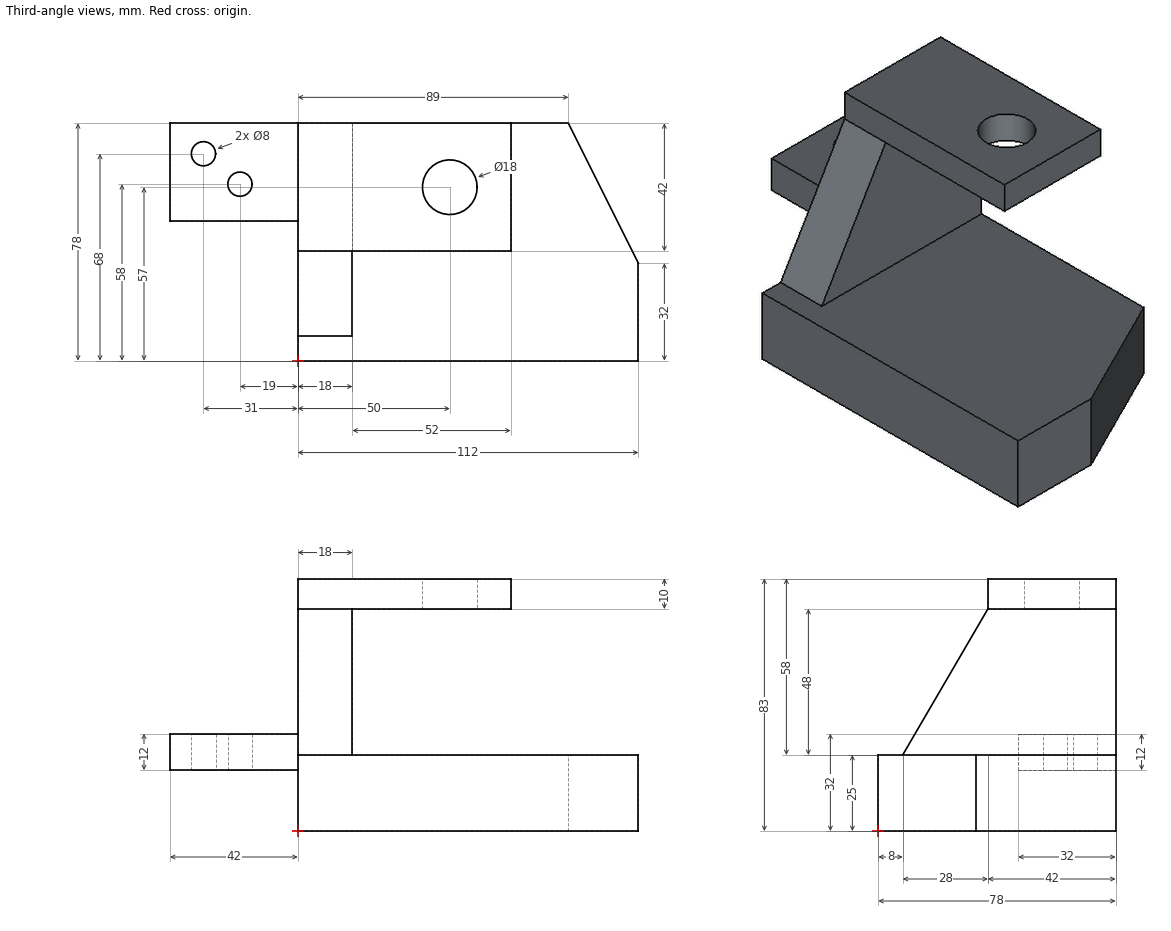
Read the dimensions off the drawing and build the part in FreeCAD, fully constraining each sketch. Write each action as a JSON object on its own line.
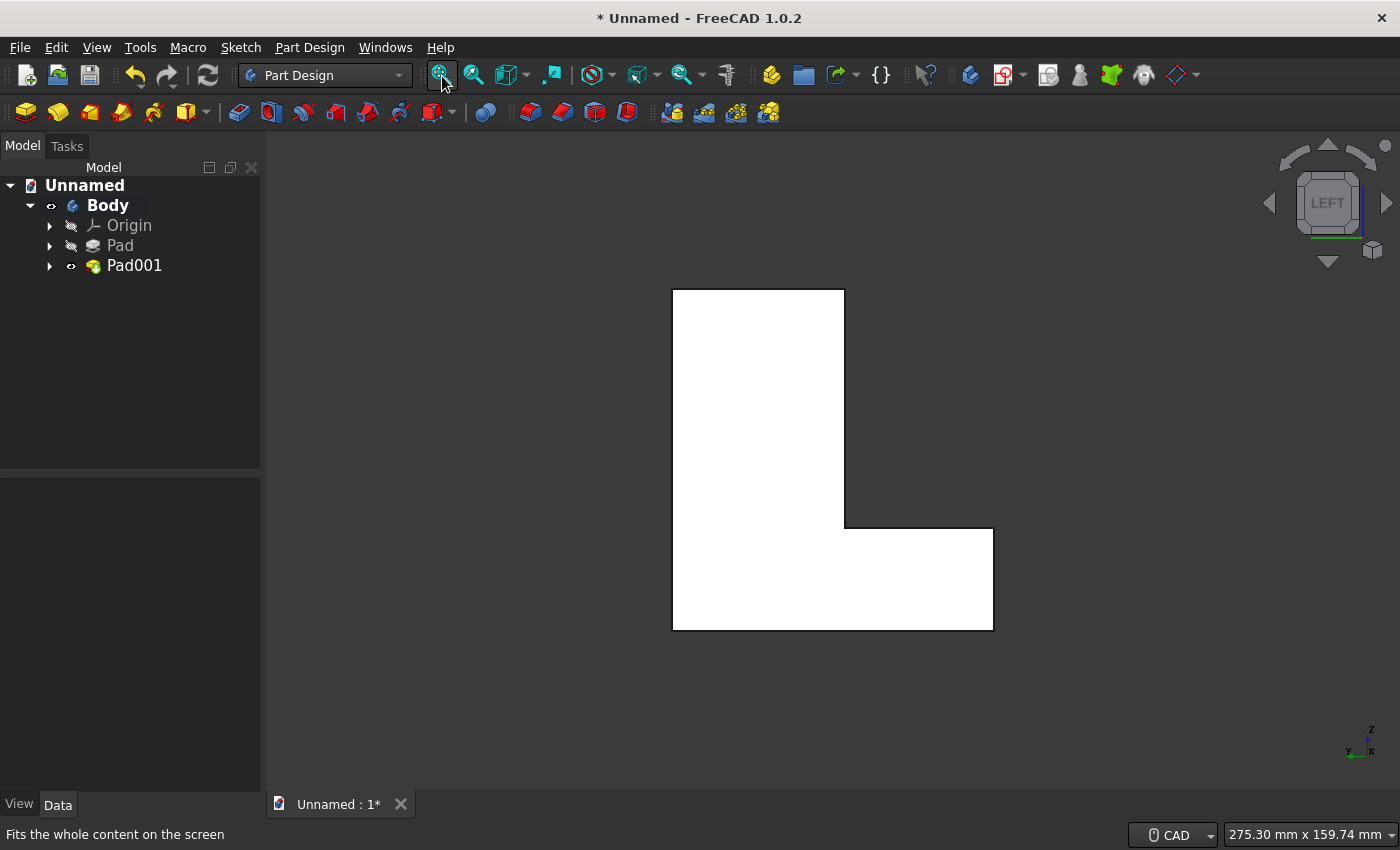
{"action": "left_click", "coordinate": [741, 361]}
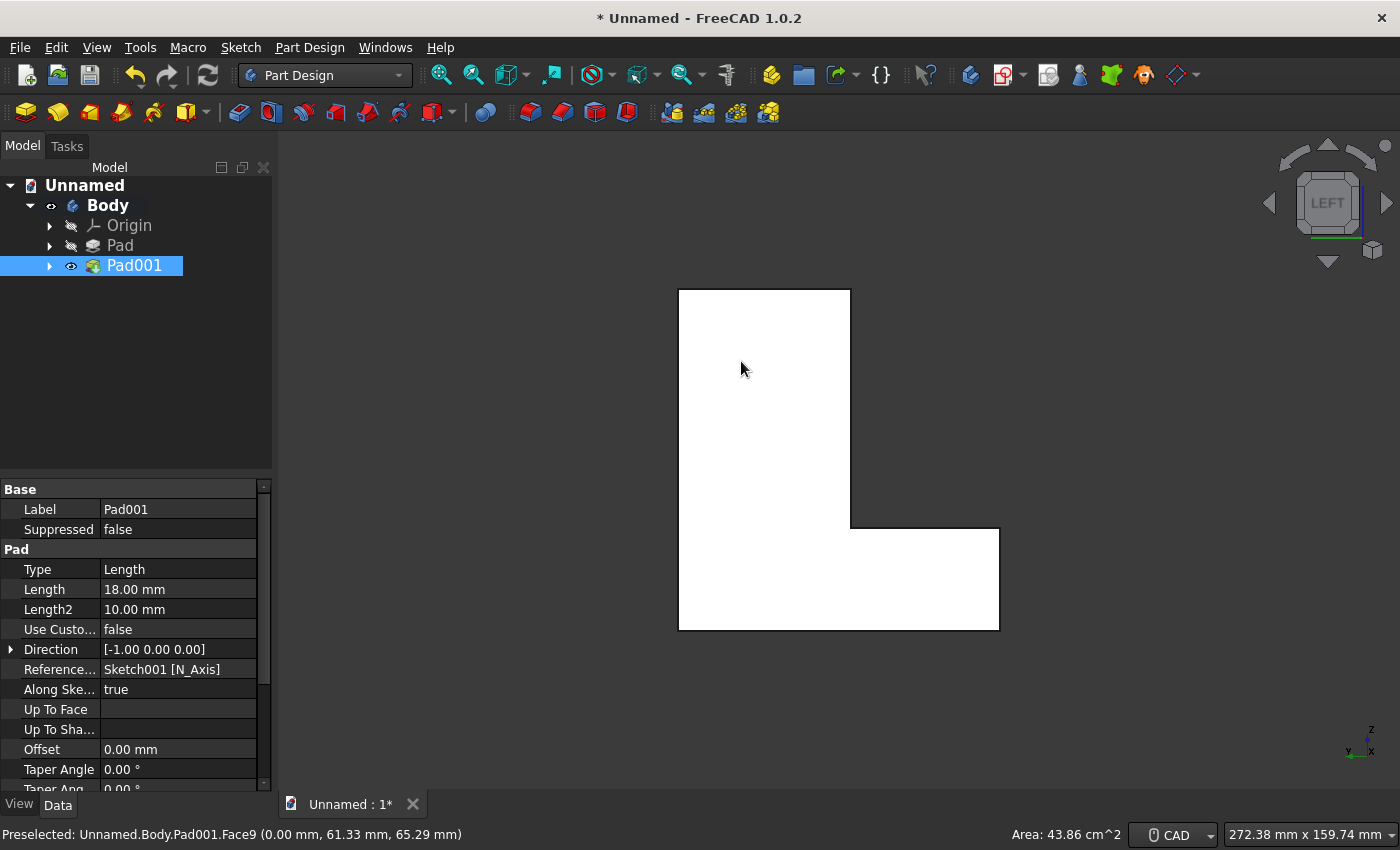
{"action": "left_click", "coordinate": [1004, 76]}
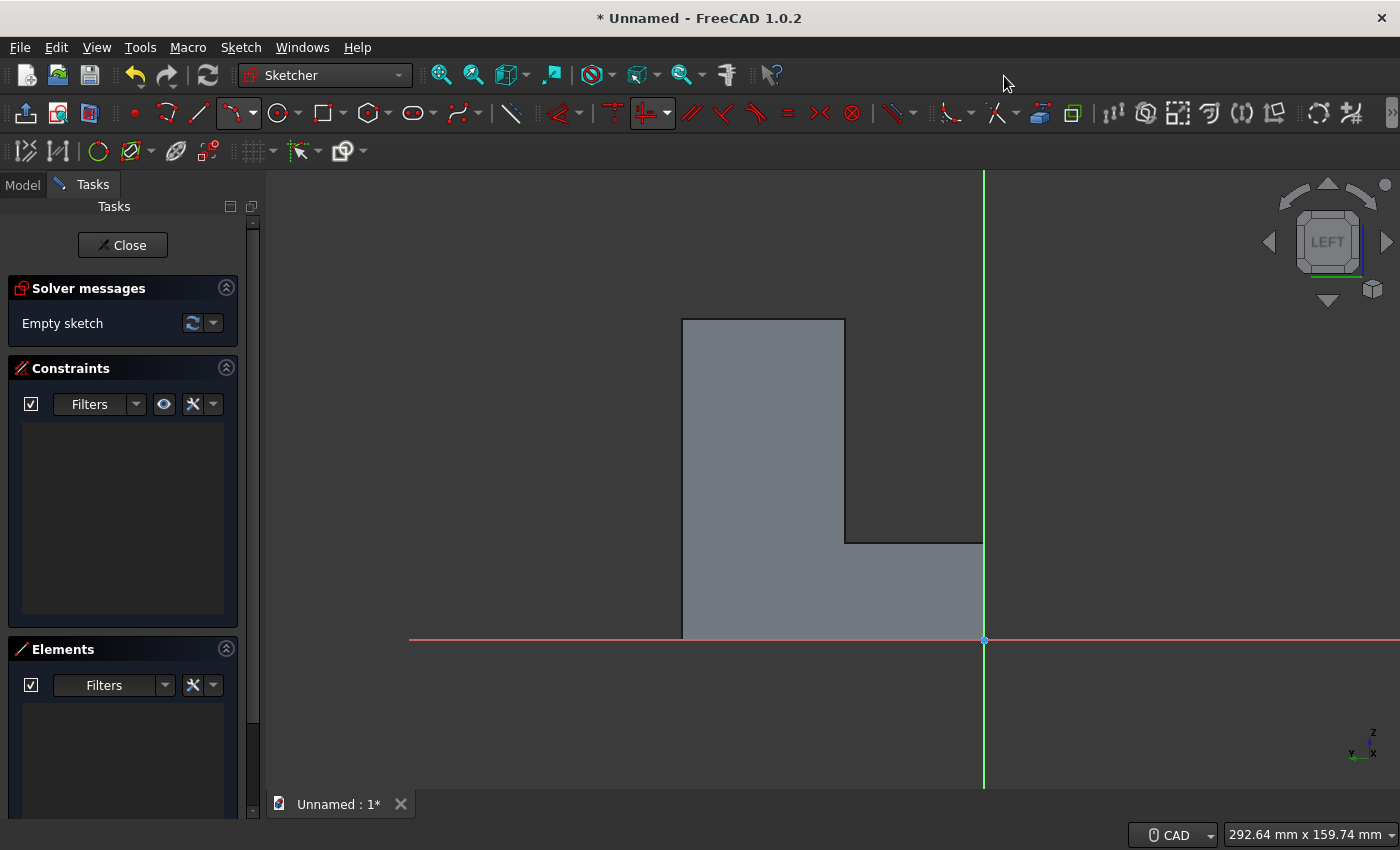
{"action": "scroll", "coordinate": [889, 659], "scroll_direction": "up", "scroll_amount": 4}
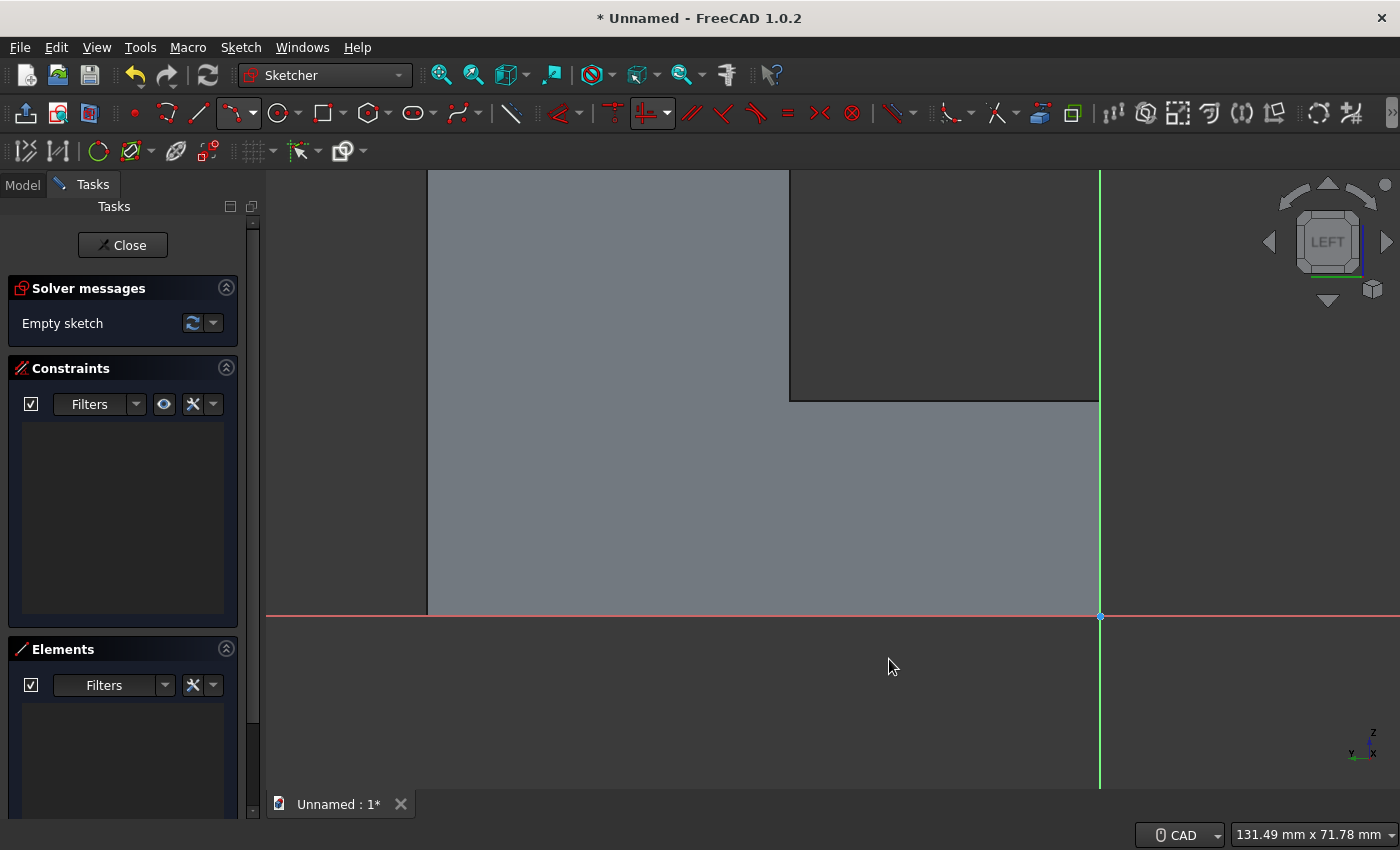
{"action": "key", "text": "g r"}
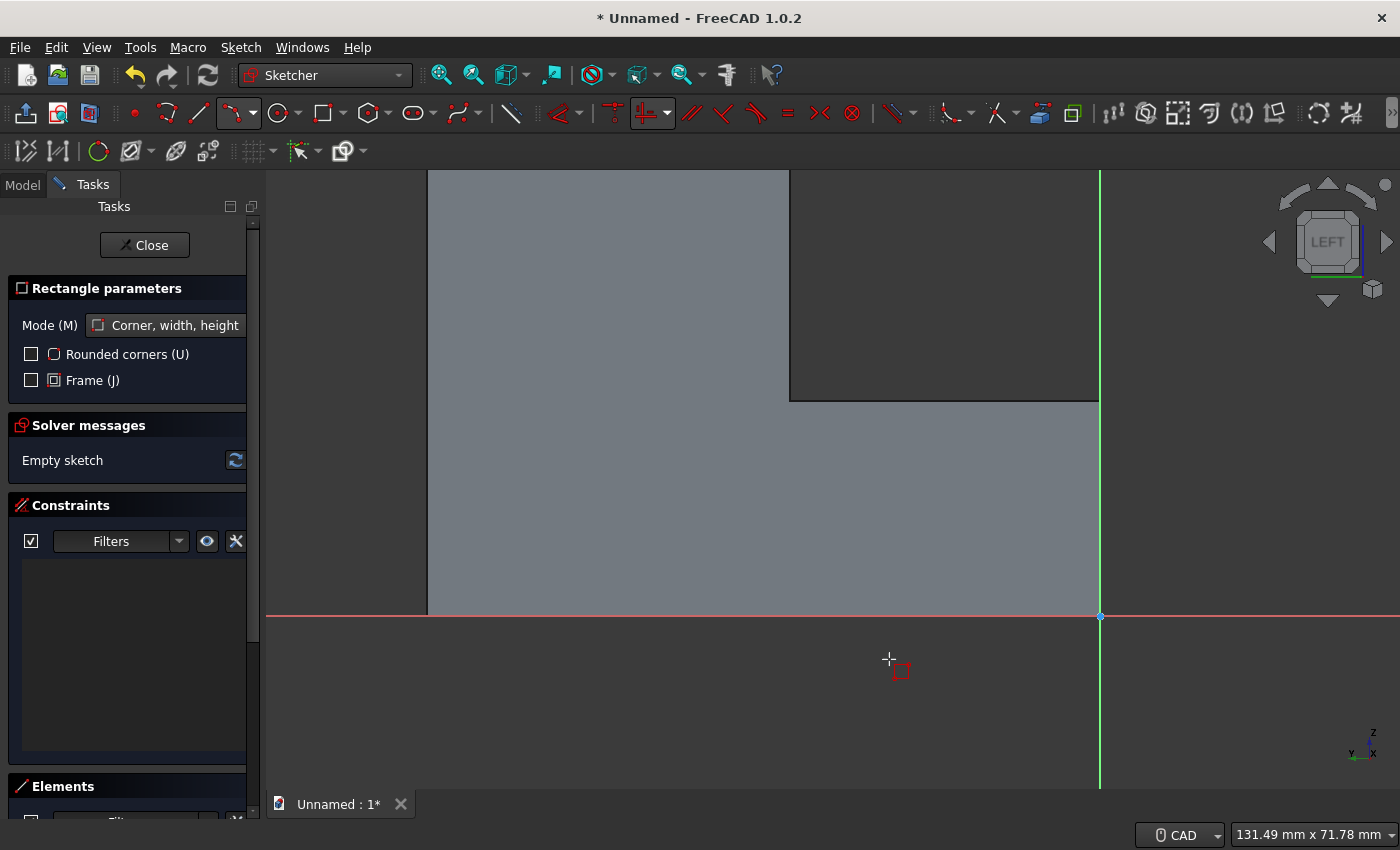
{"action": "left_click", "coordinate": [427, 340]}
{"action": "mouse_move", "coordinate": [703, 444]}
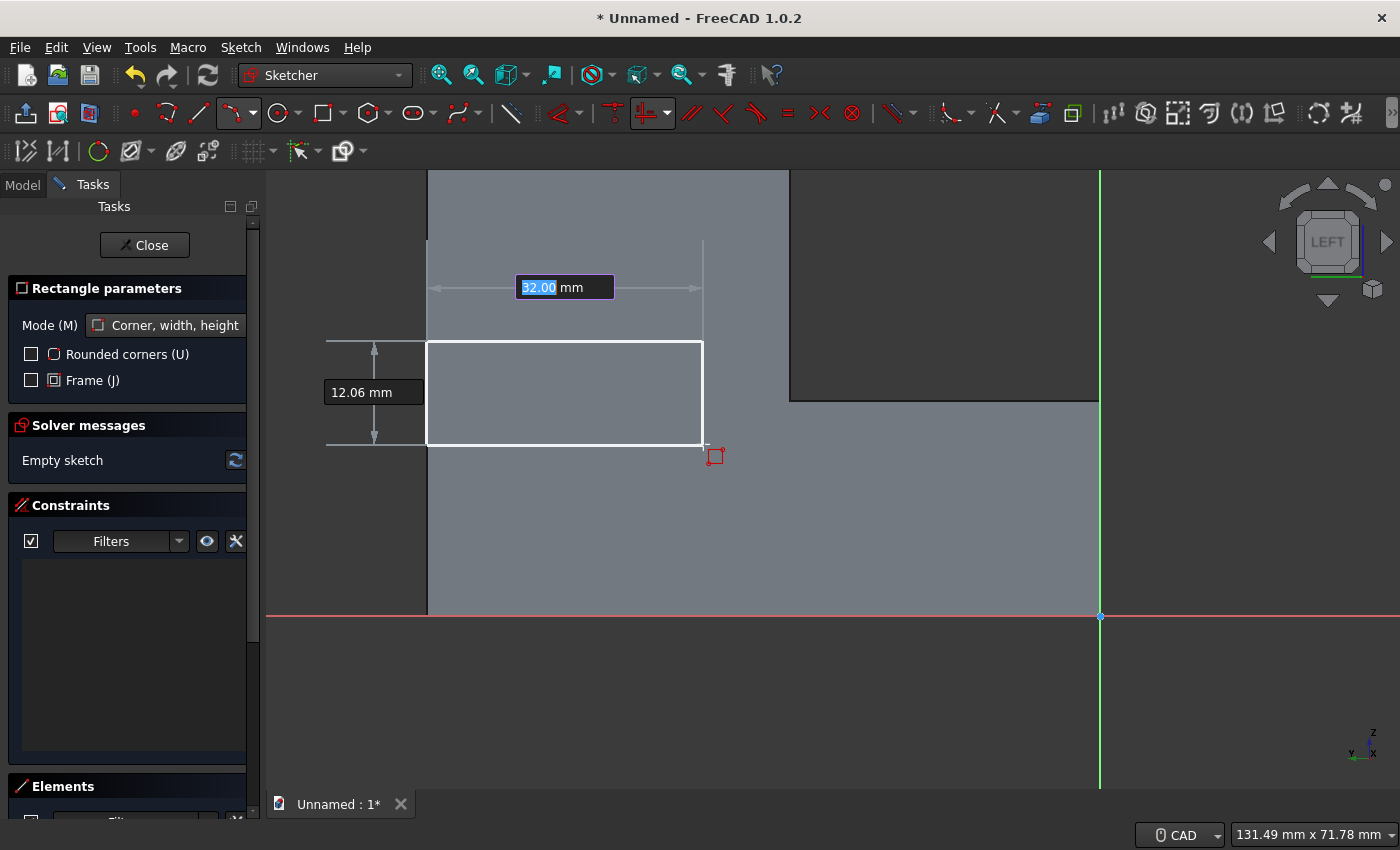
{"action": "type", "text": "32"}
{"action": "key", "text": "Tab"}
{"action": "type", "text": "12"}
{"action": "key", "text": "Return"}
{"action": "key", "text": "Escape"}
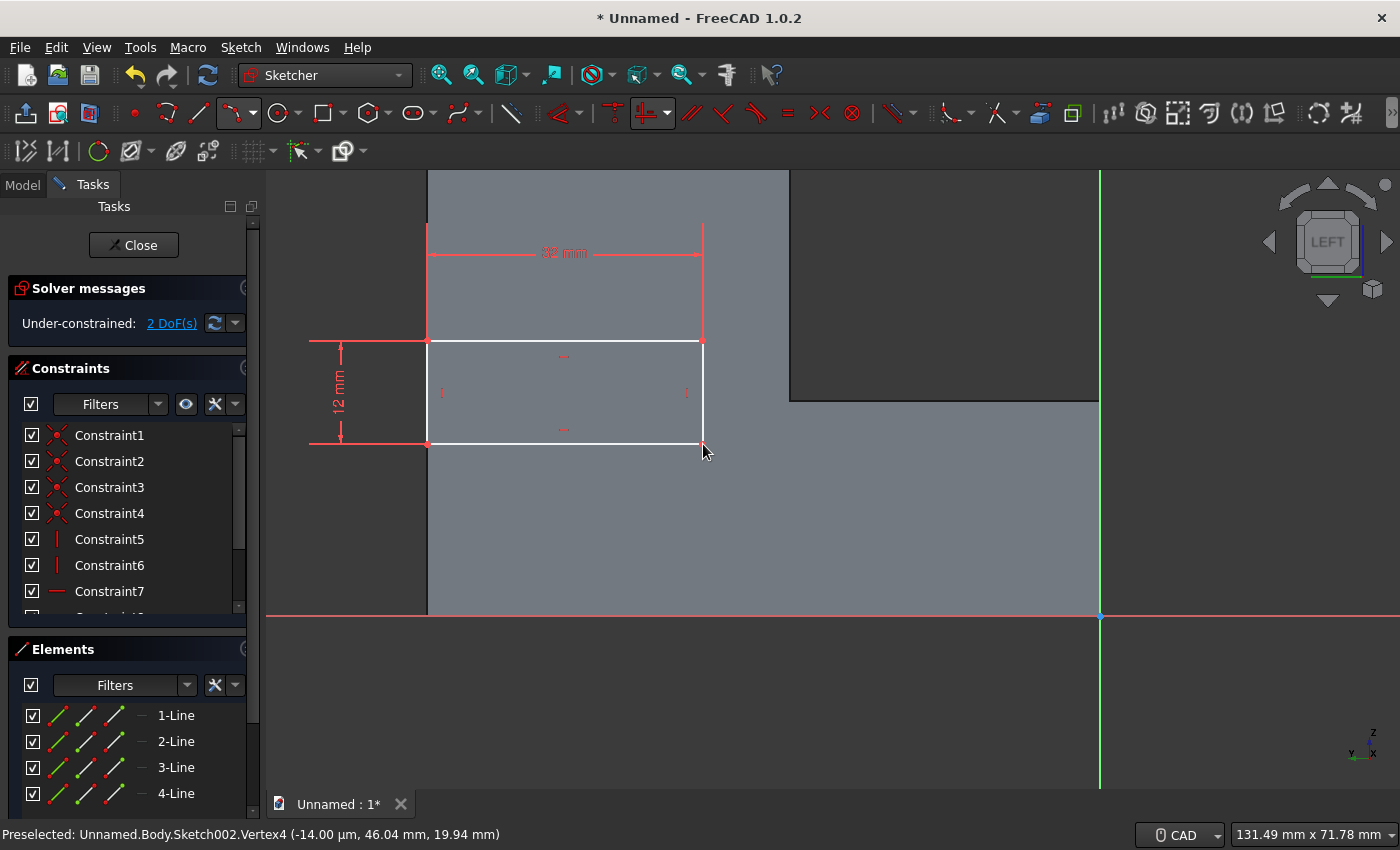
{"action": "key", "text": "d"}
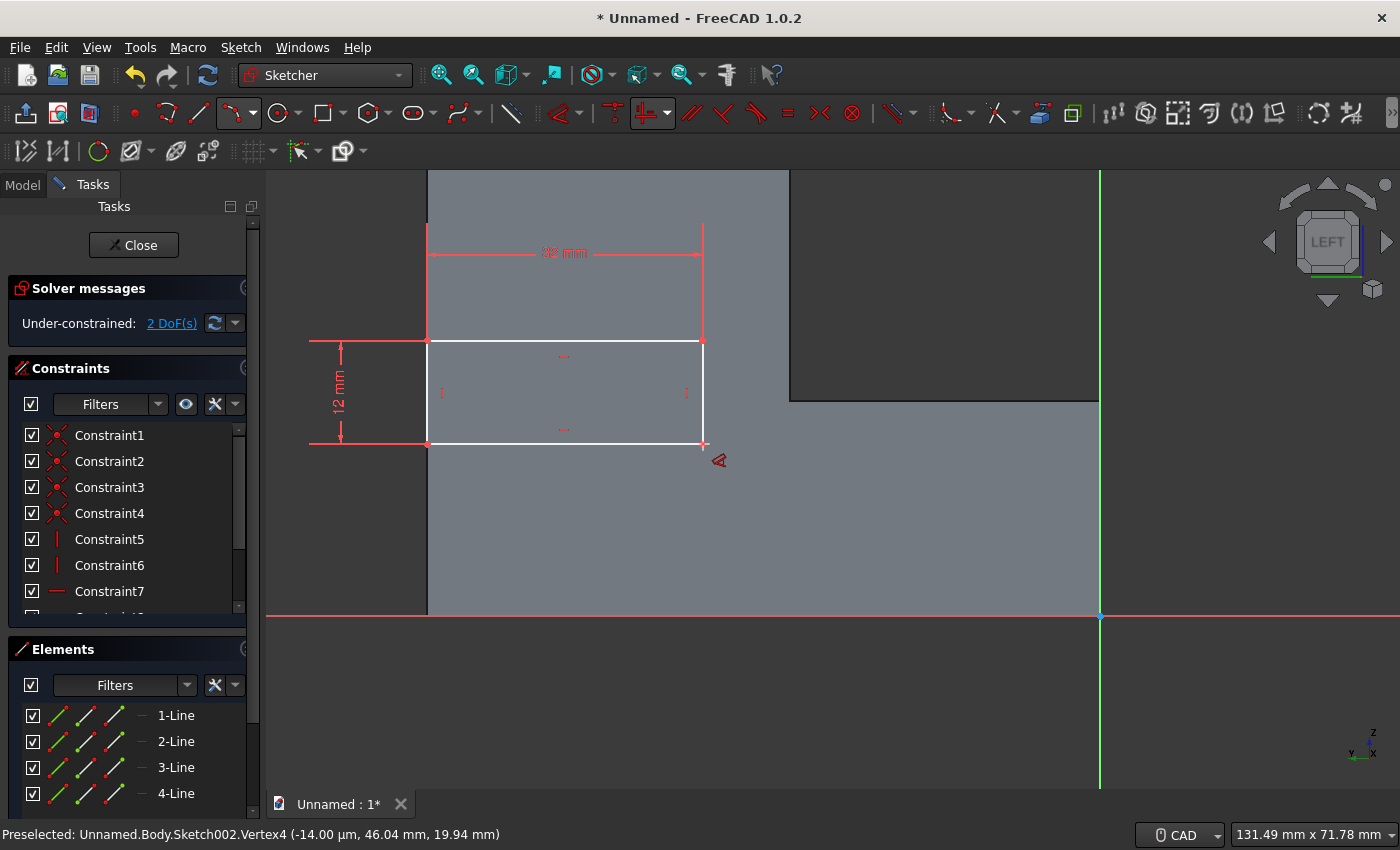
{"action": "left_click", "coordinate": [427, 341]}
{"action": "left_click", "coordinate": [764, 650]}